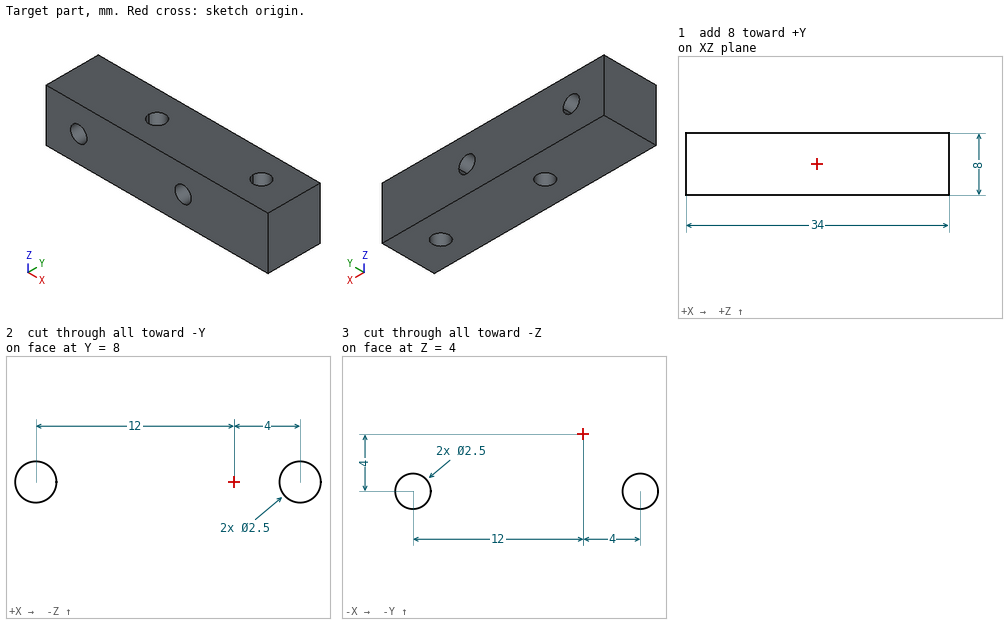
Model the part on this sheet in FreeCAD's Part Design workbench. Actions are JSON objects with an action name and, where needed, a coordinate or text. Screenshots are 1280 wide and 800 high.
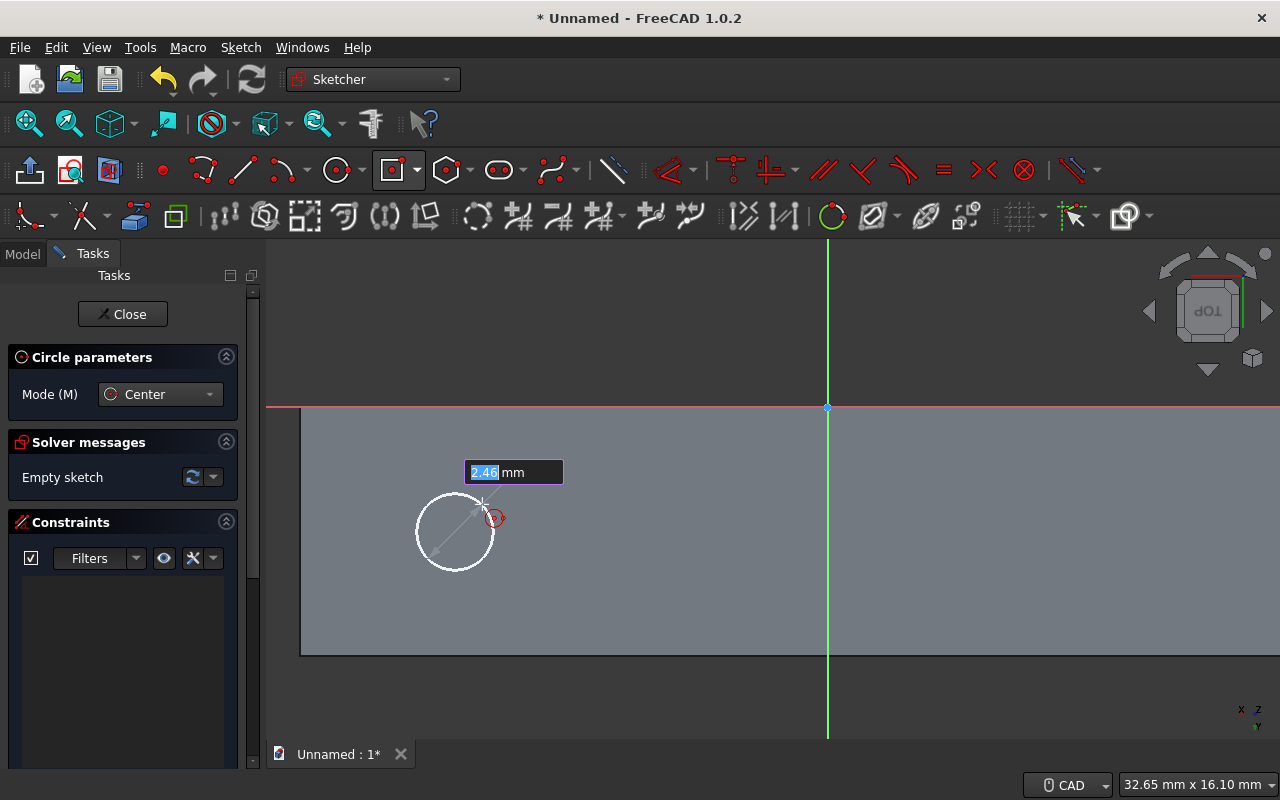
{"action": "type", "text": "2.5"}
{"action": "key", "text": "Return"}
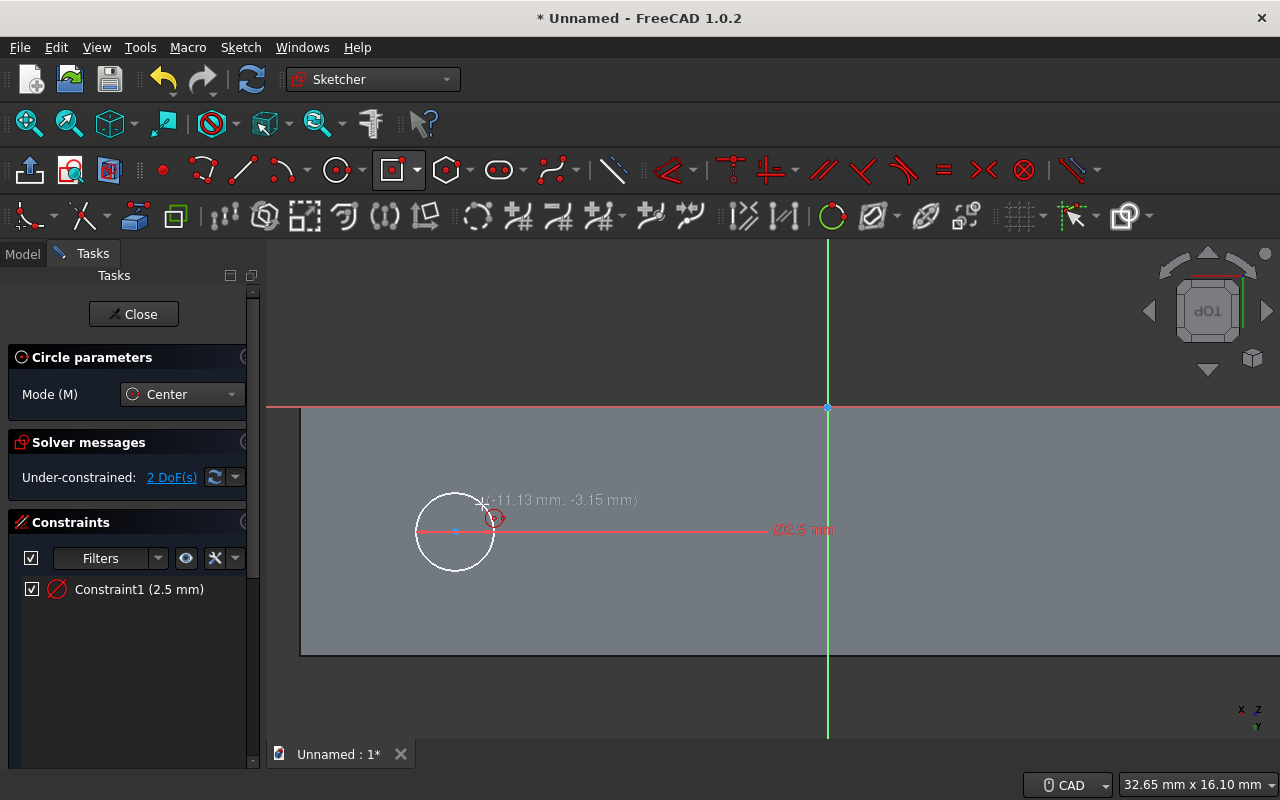
{"action": "left_click", "coordinate": [952, 531]}
{"action": "mouse_move", "coordinate": [979, 504]}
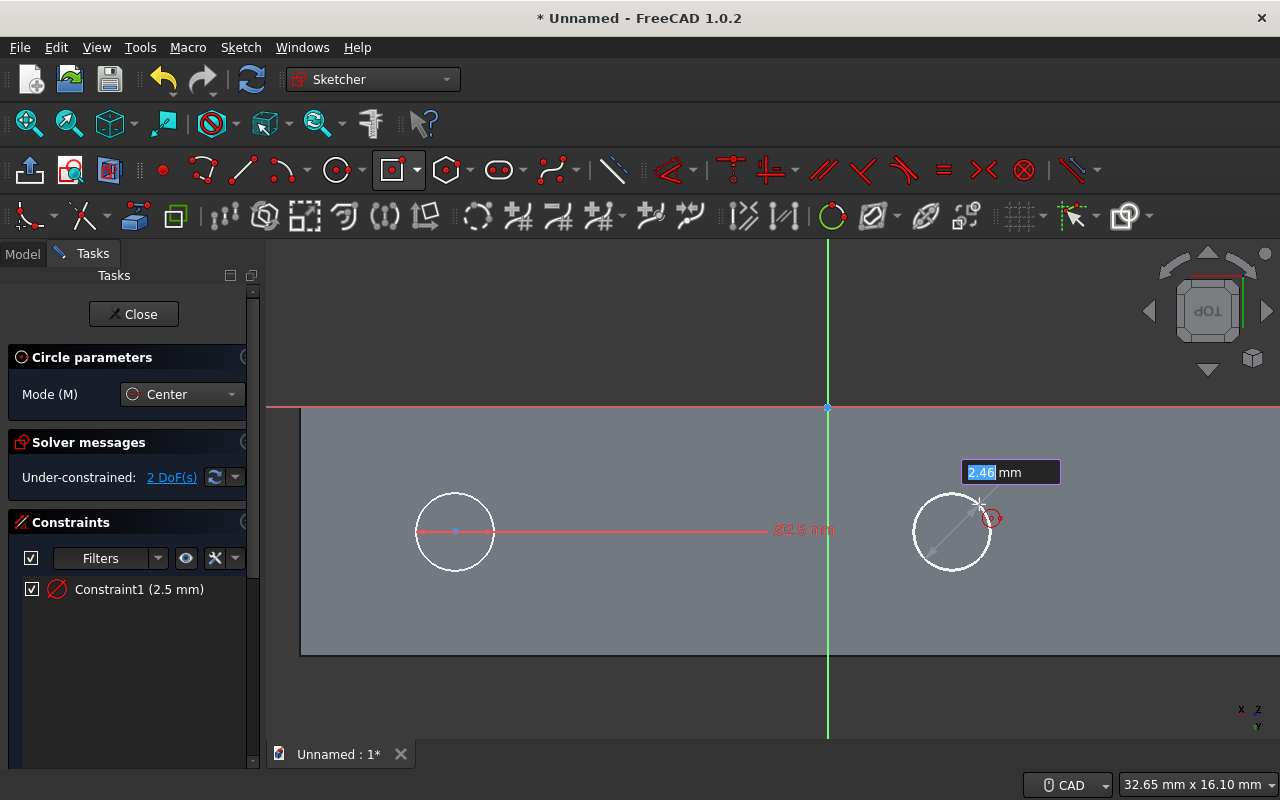
{"action": "type", "text": "2.5"}
{"action": "key", "text": "Return"}
{"action": "key", "text": "Escape"}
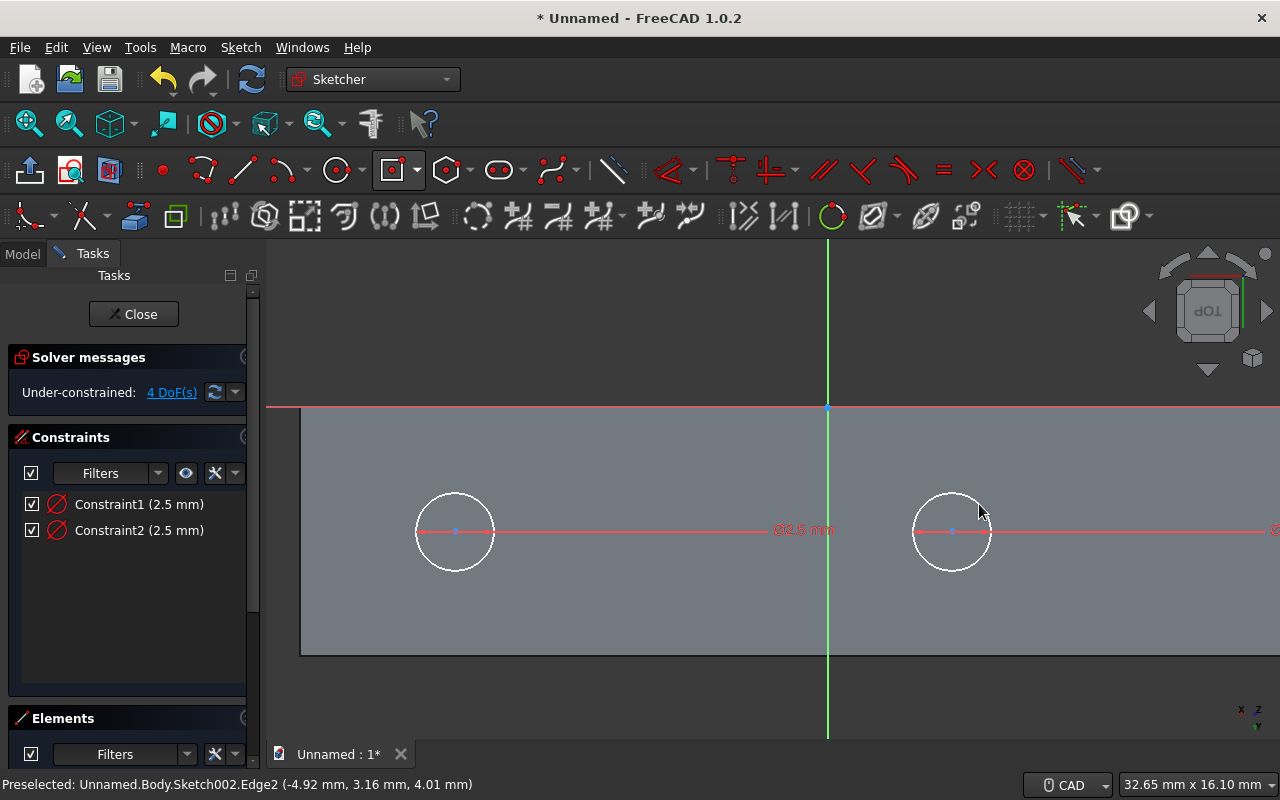
{"action": "left_click", "coordinate": [455, 532]}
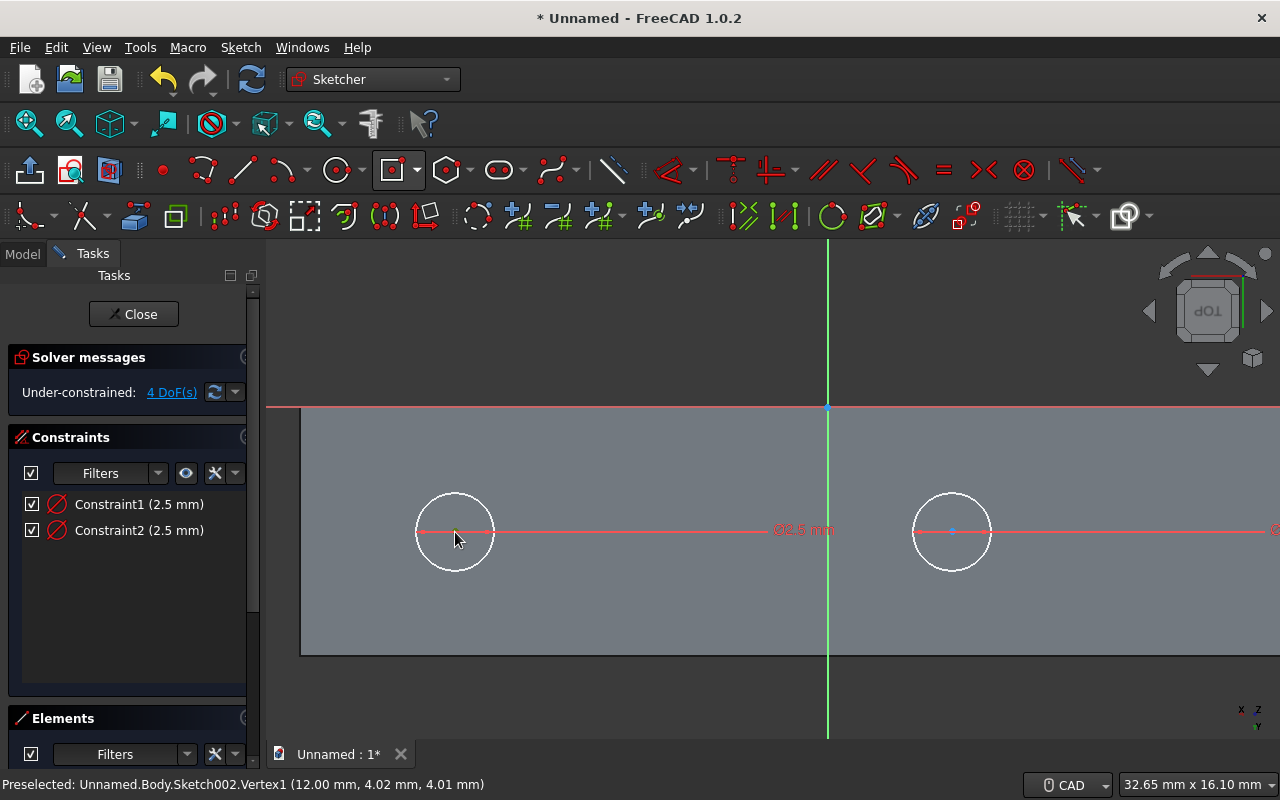
{"action": "left_click", "coordinate": [952, 532]}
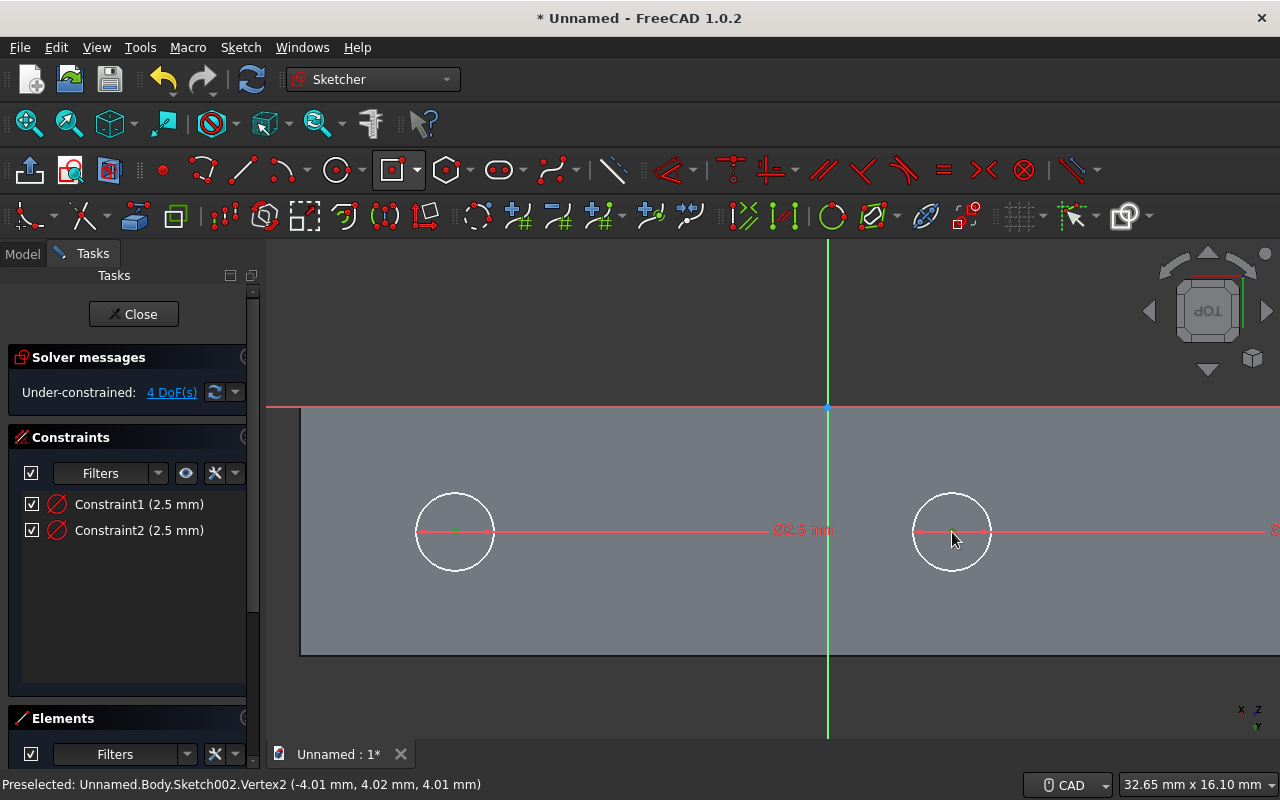
{"action": "left_click", "coordinate": [798, 170]}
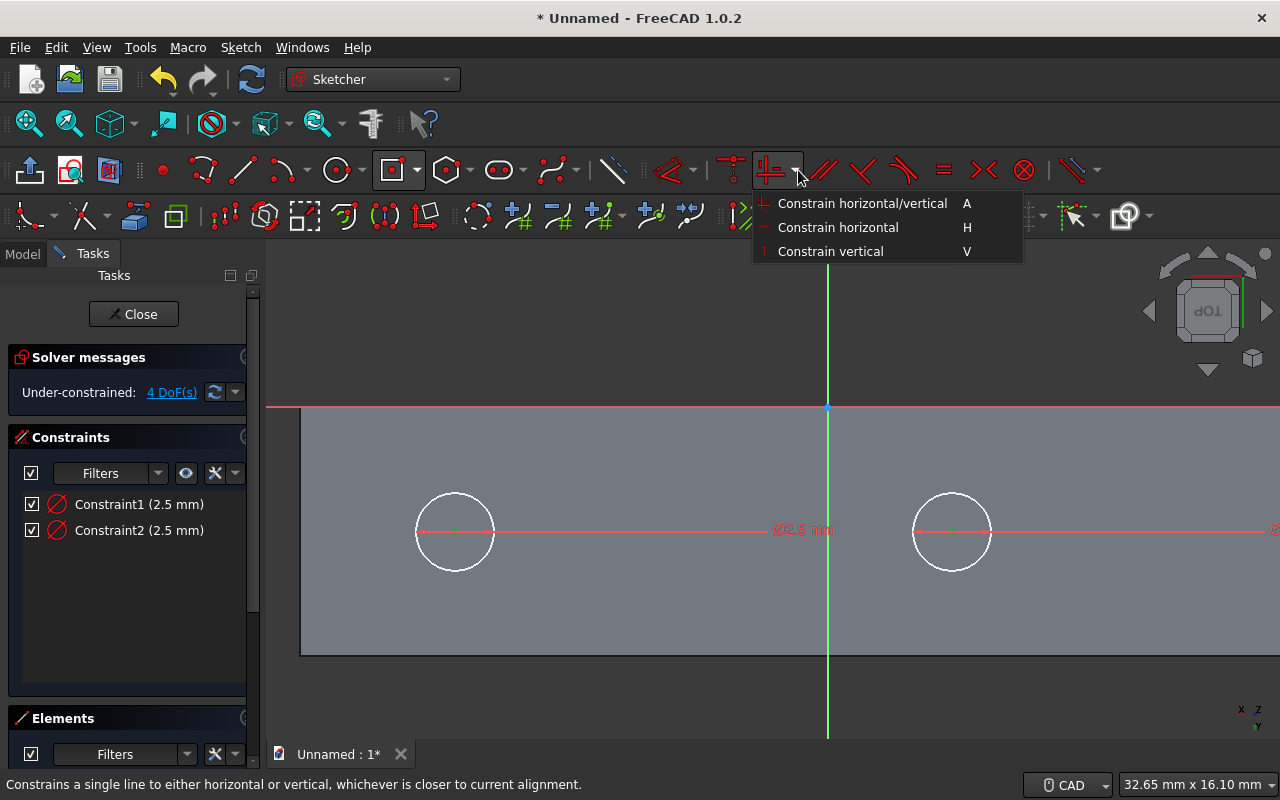
{"action": "left_click", "coordinate": [888, 227]}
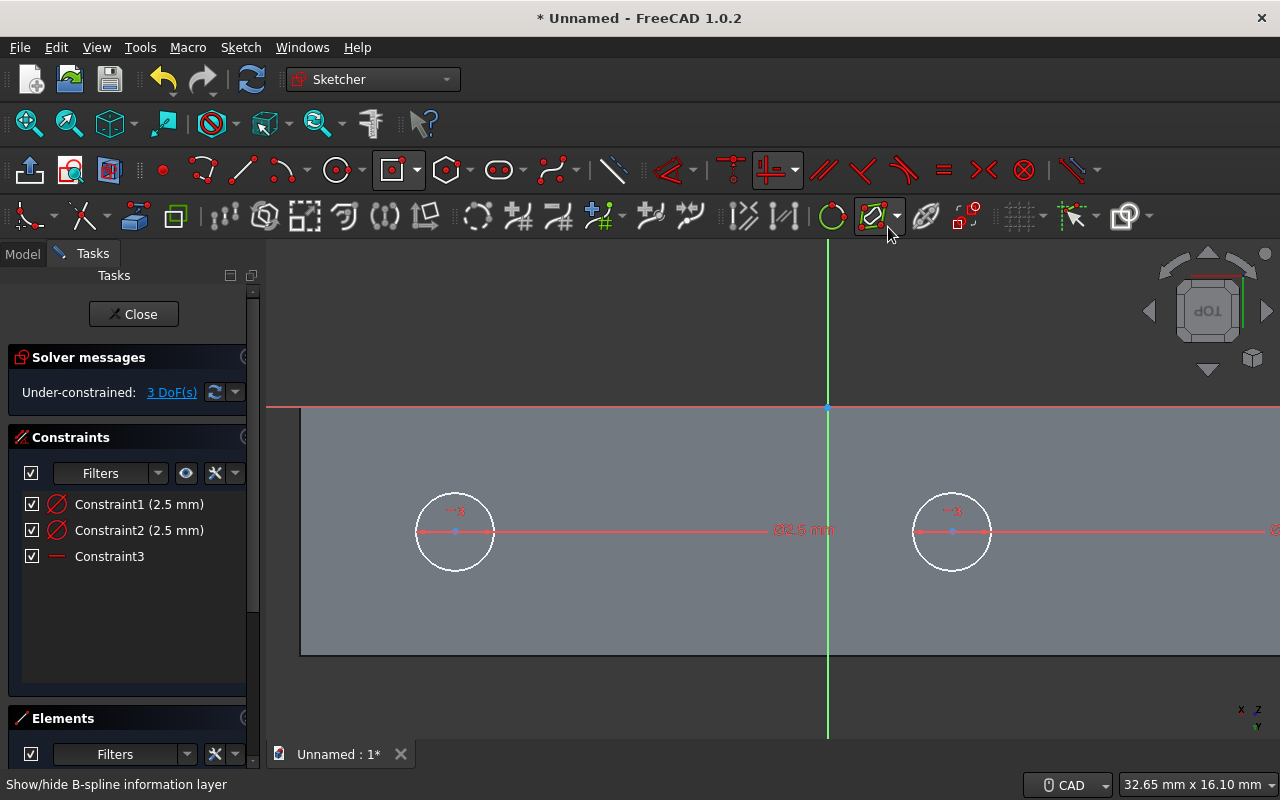
{"action": "left_click", "coordinate": [668, 170]}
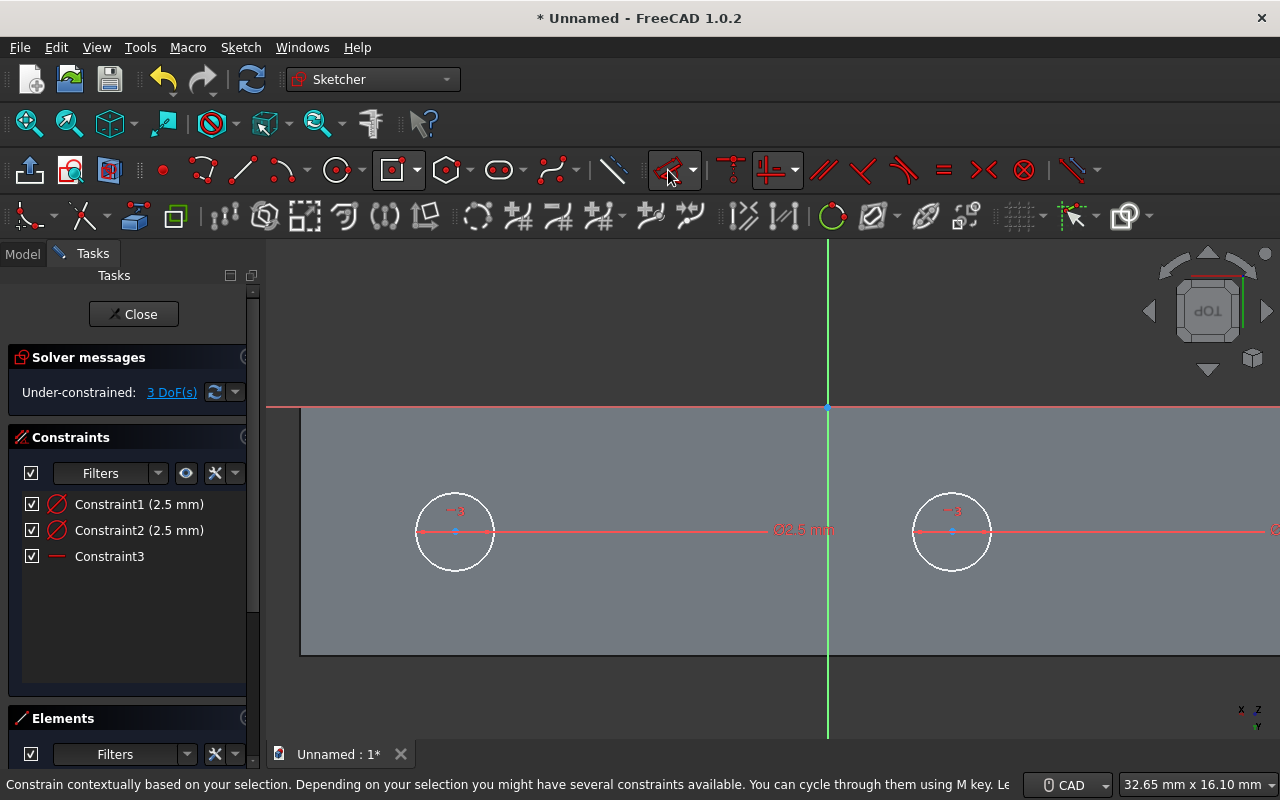
{"action": "left_click", "coordinate": [455, 532]}
{"action": "left_click", "coordinate": [421, 470]}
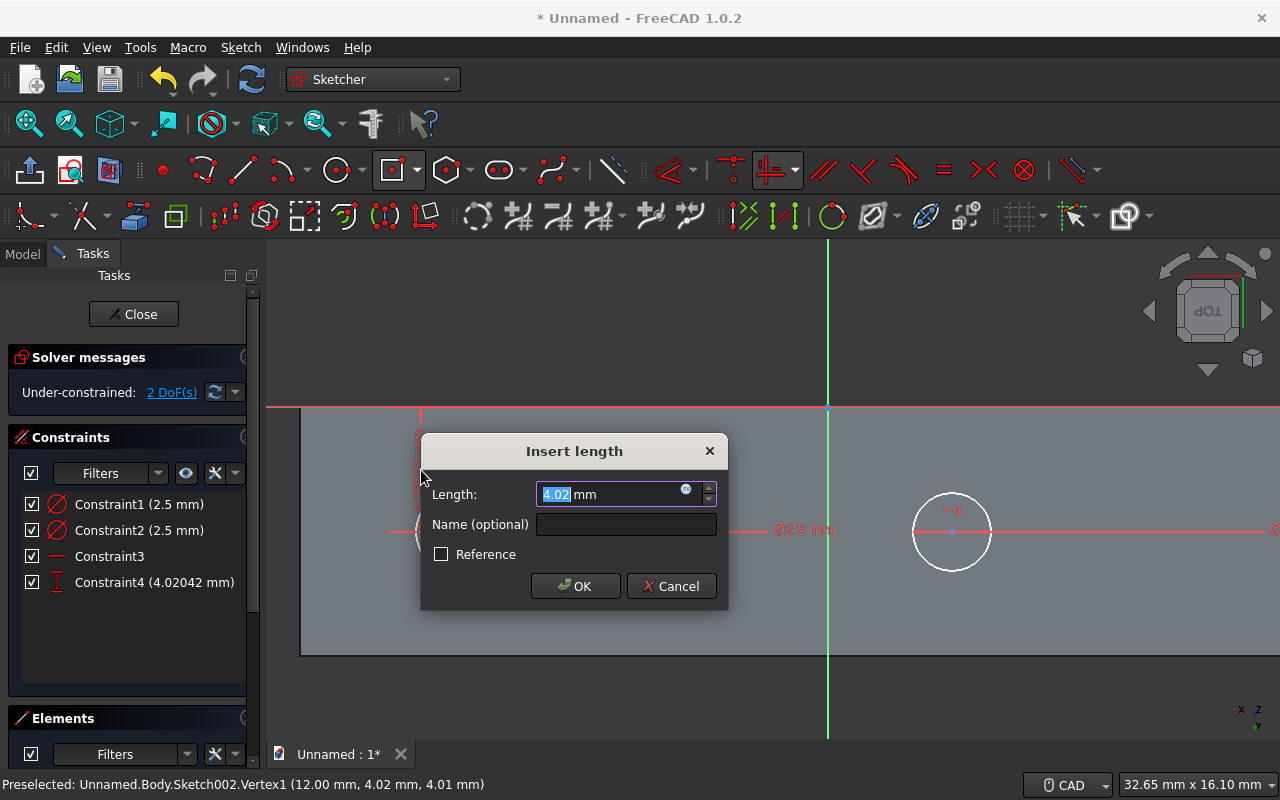
{"action": "type", "text": "4"}
{"action": "key", "text": "Return"}